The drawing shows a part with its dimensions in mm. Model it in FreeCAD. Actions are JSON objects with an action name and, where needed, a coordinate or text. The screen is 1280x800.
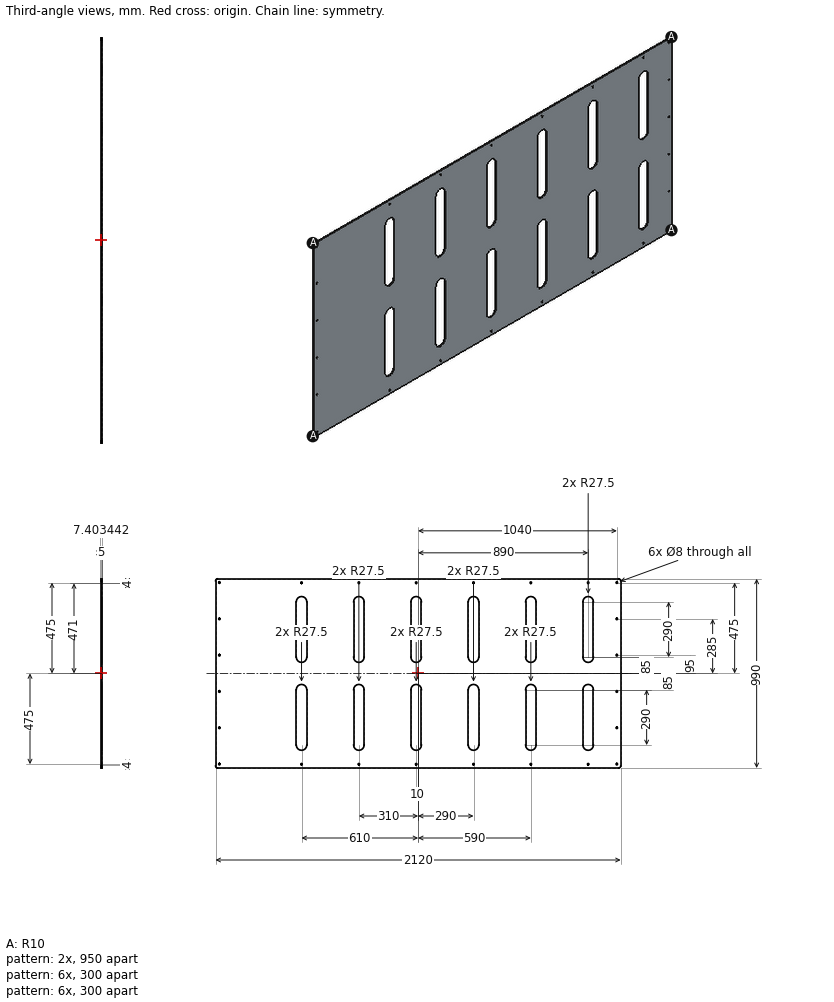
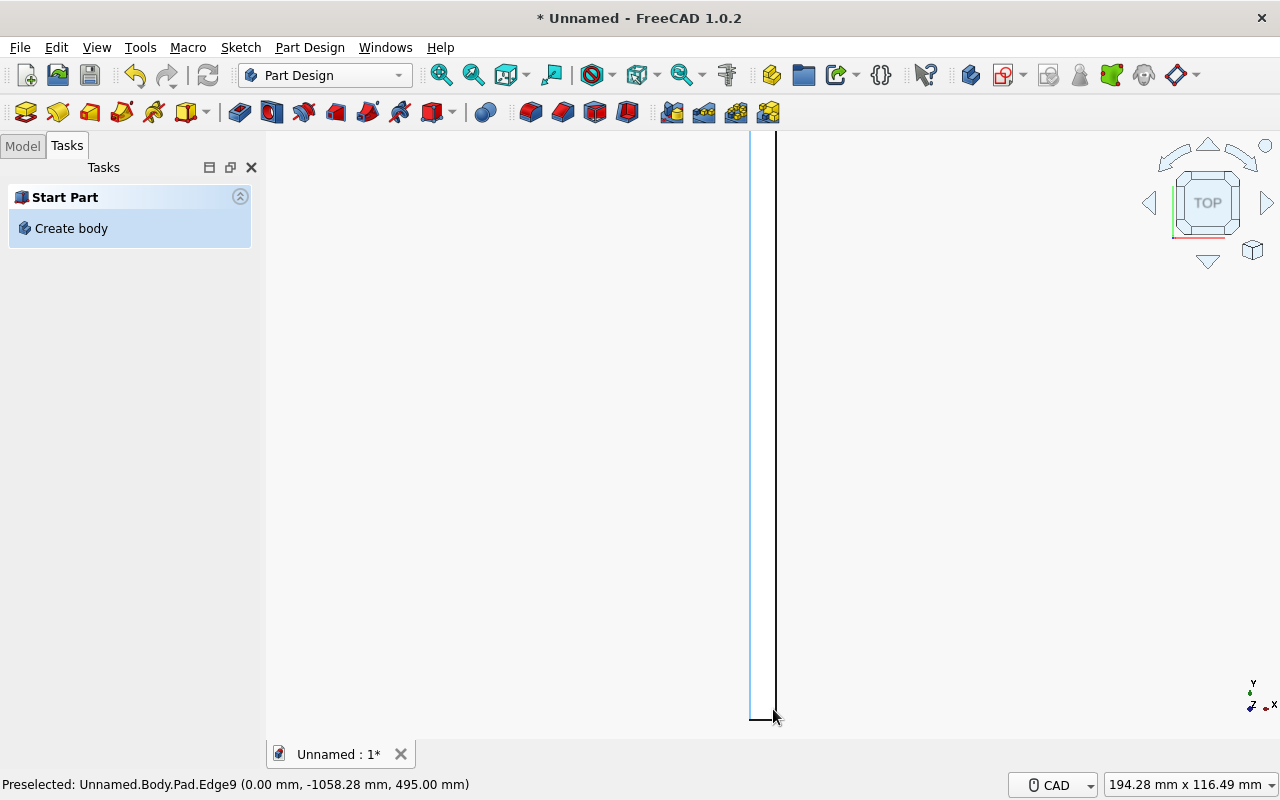
{"action": "left_click", "coordinate": [442, 76]}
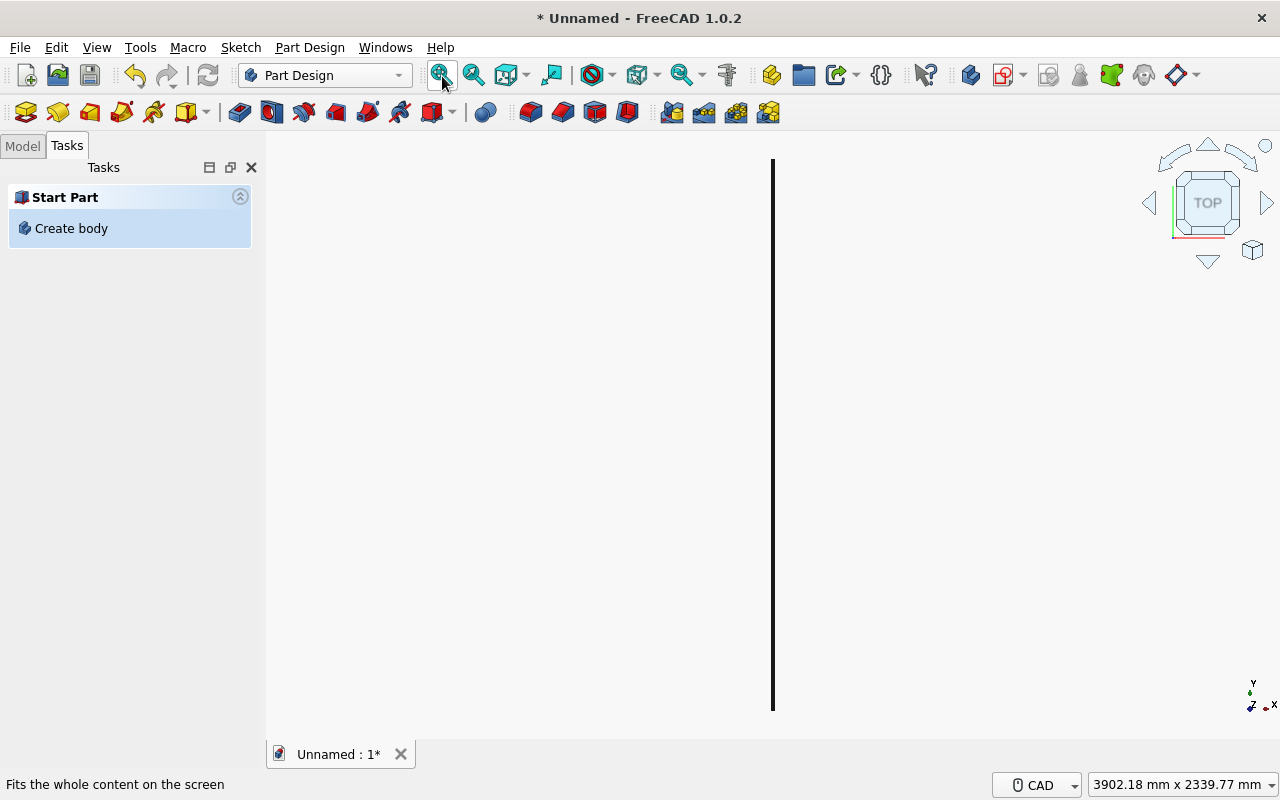
{"action": "key", "text": "1"}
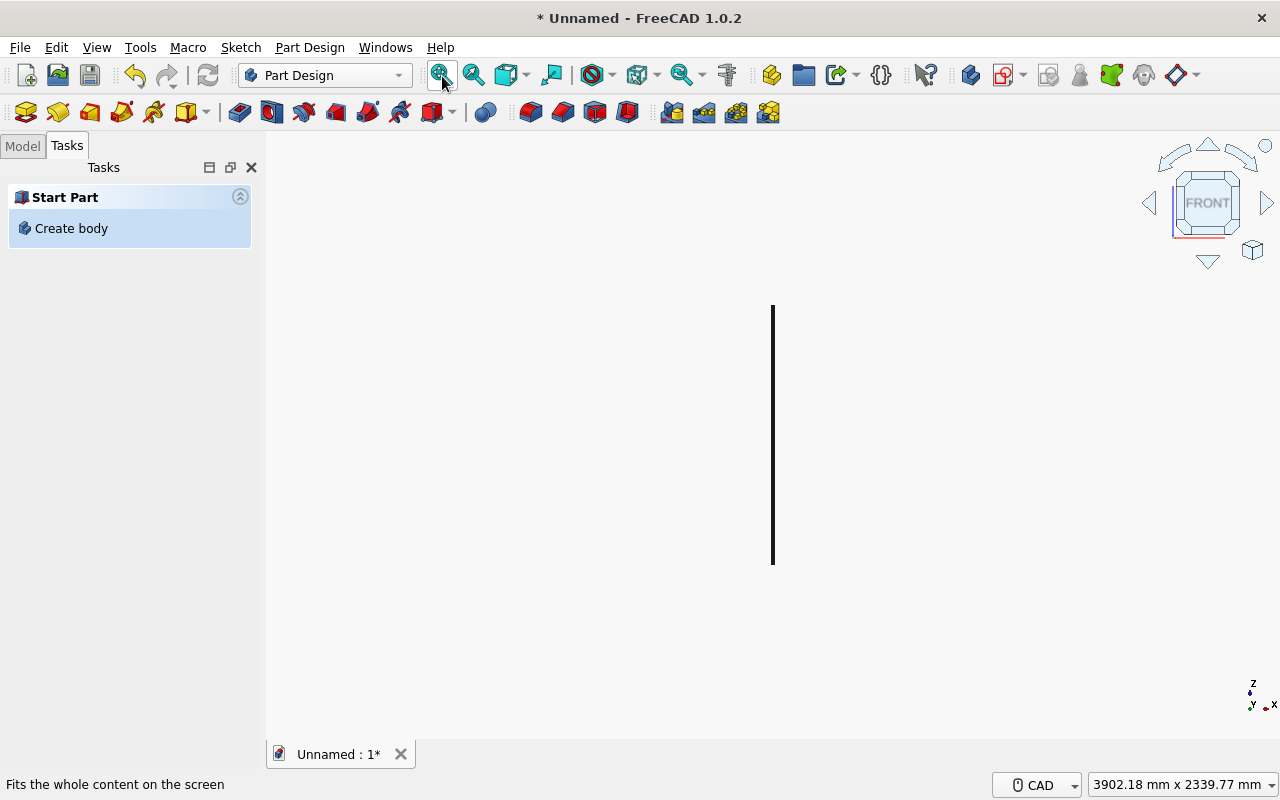
{"action": "key", "text": "v f"}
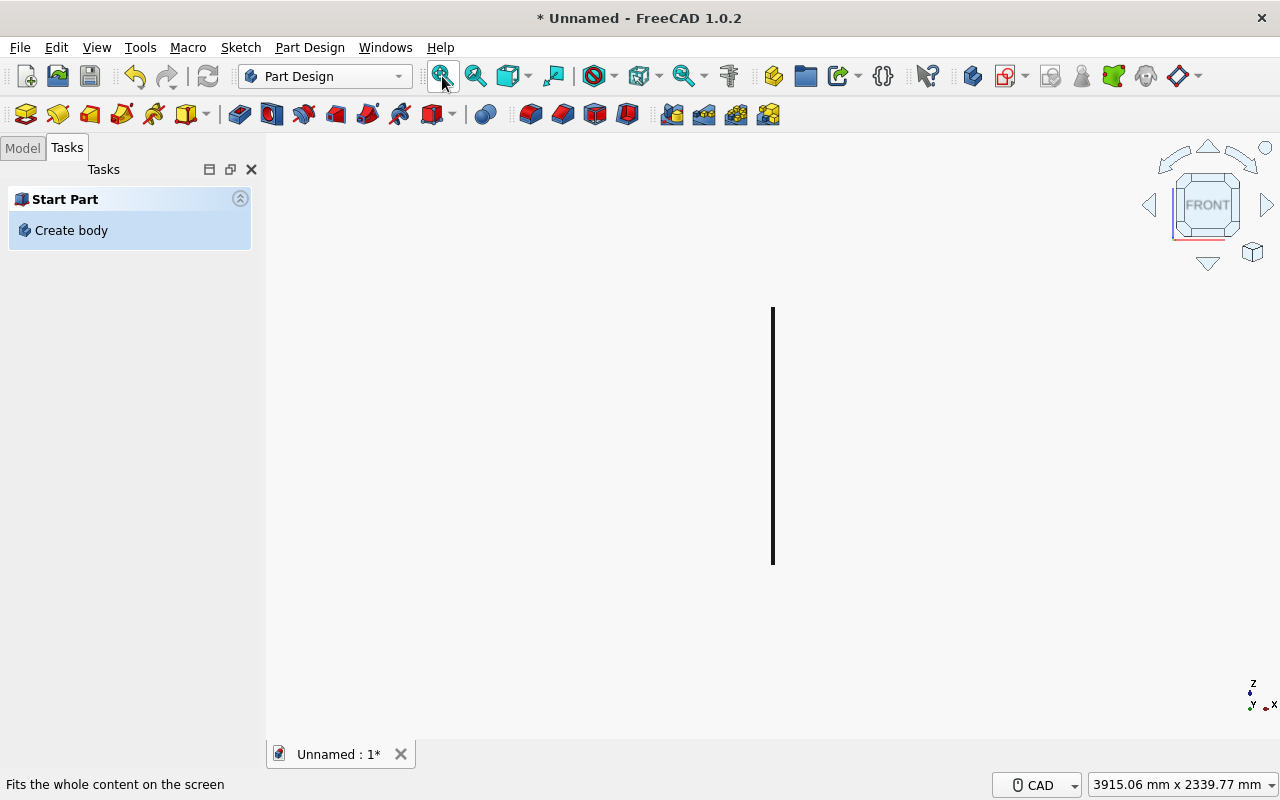
{"action": "scroll", "coordinate": [773, 563], "scroll_direction": "up", "scroll_amount": 15}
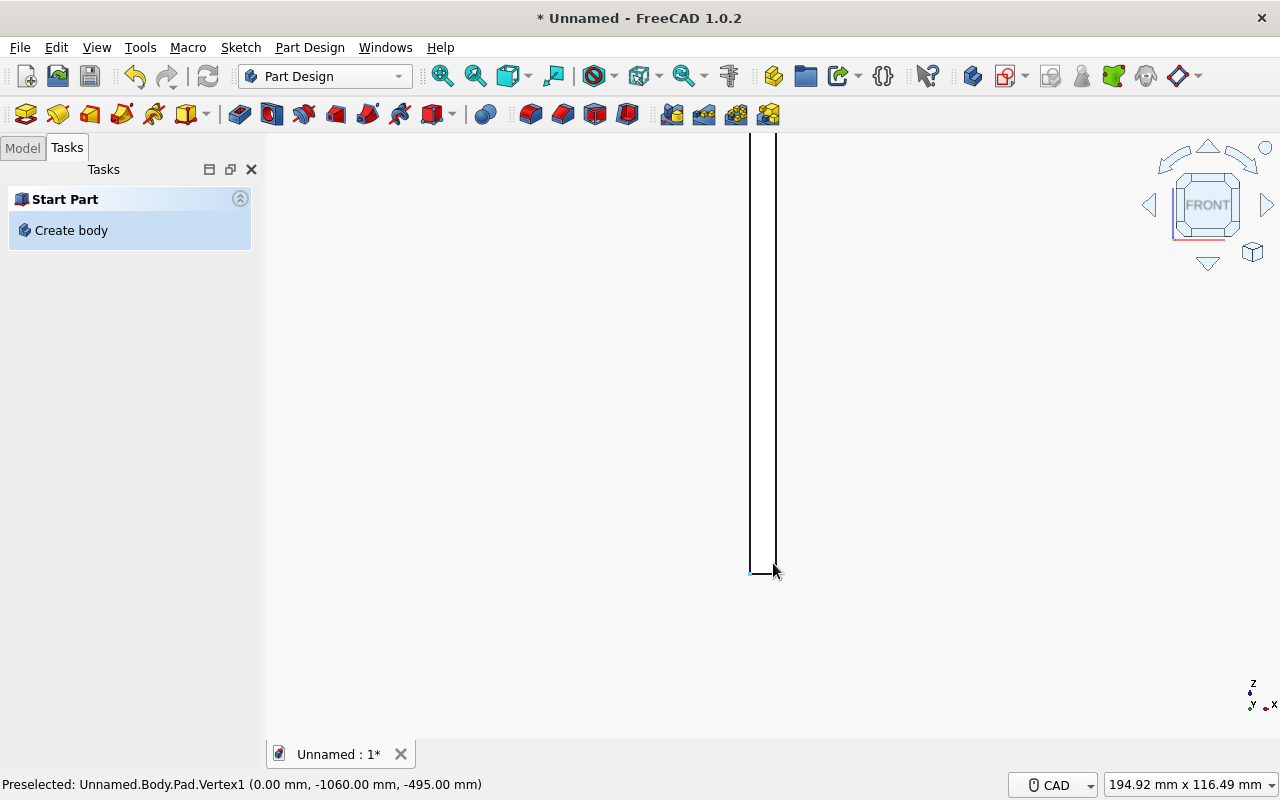
{"action": "left_click", "coordinate": [763, 573]}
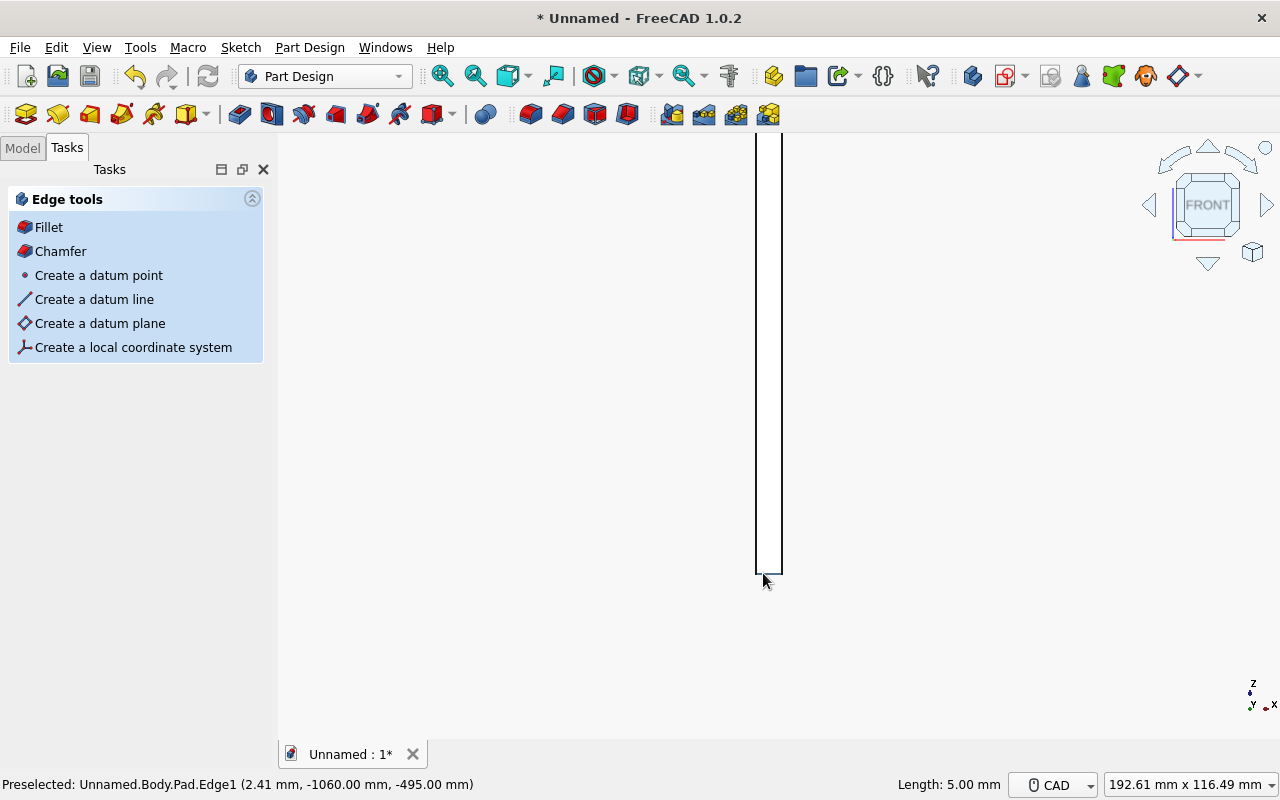
{"action": "left_click", "coordinate": [444, 76]}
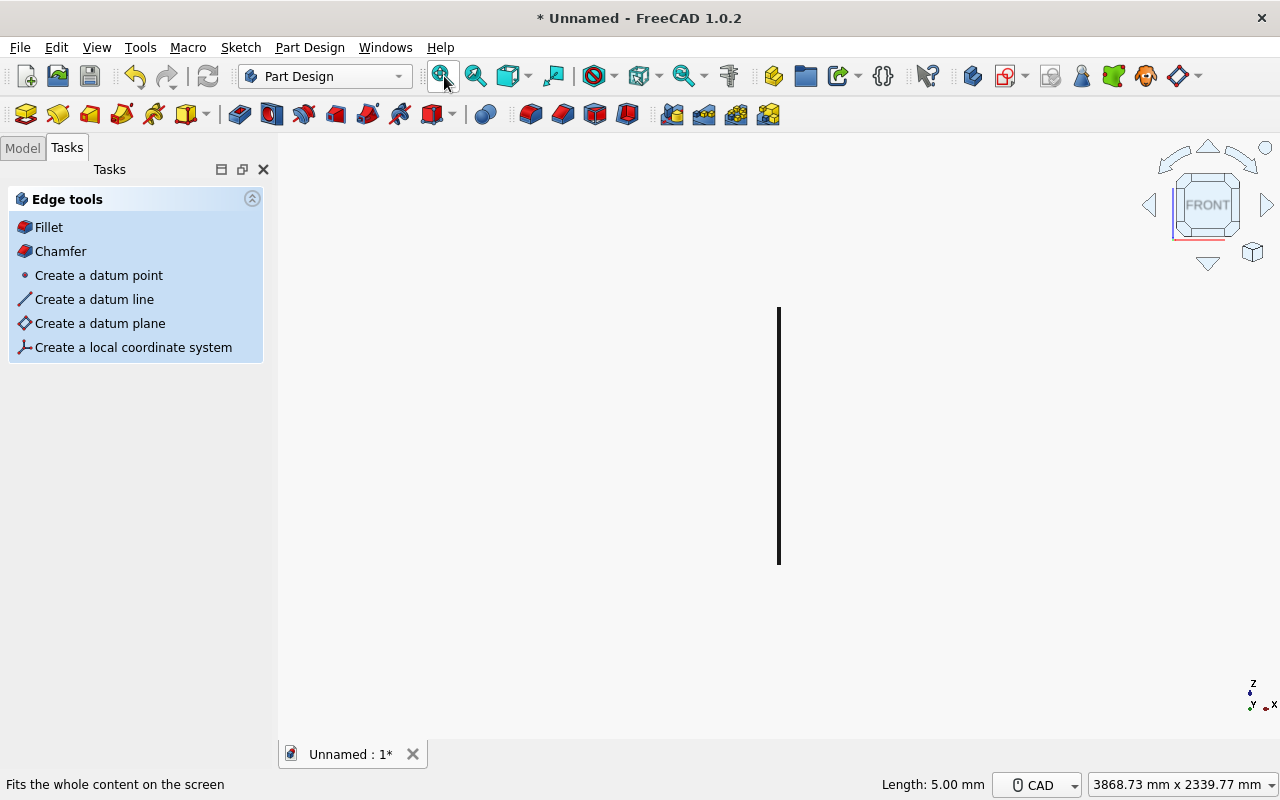
{"action": "key", "text": "3"}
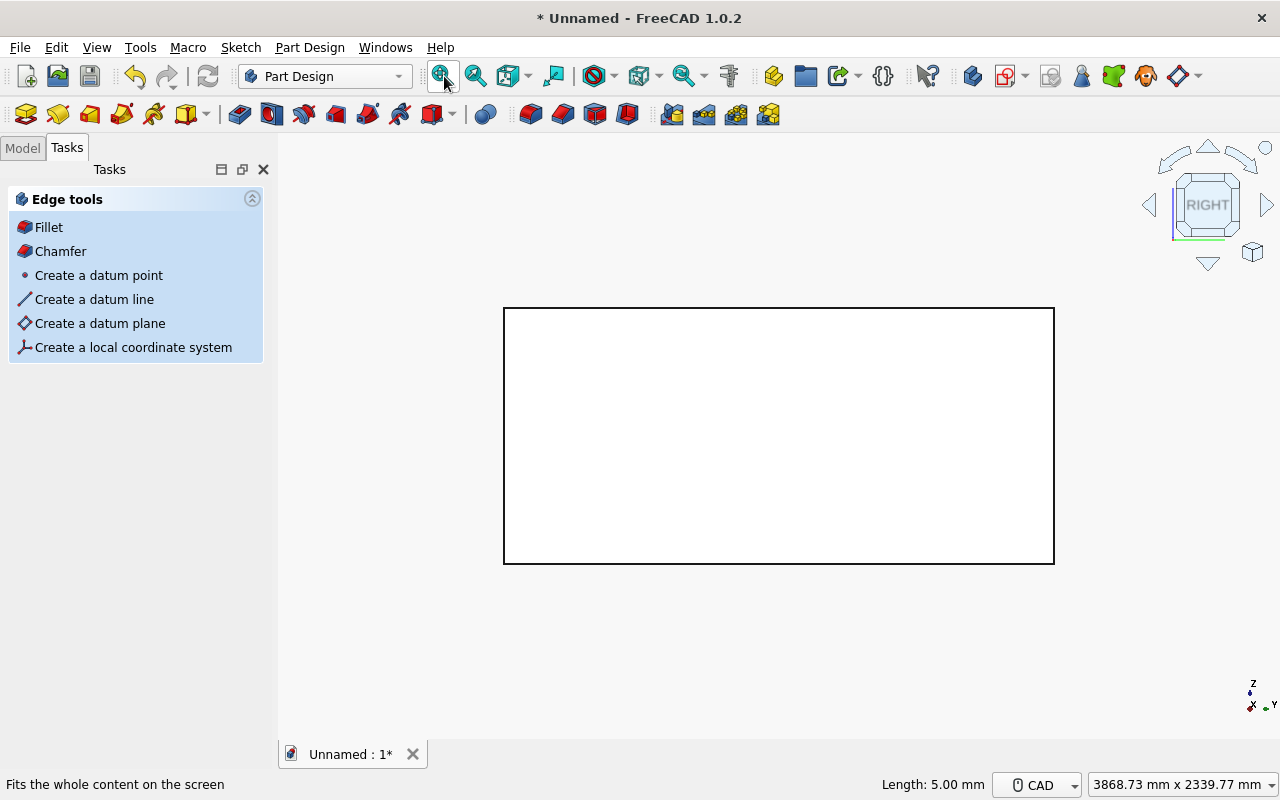
{"action": "scroll", "coordinate": [504, 307], "scroll_direction": "up", "scroll_amount": 15}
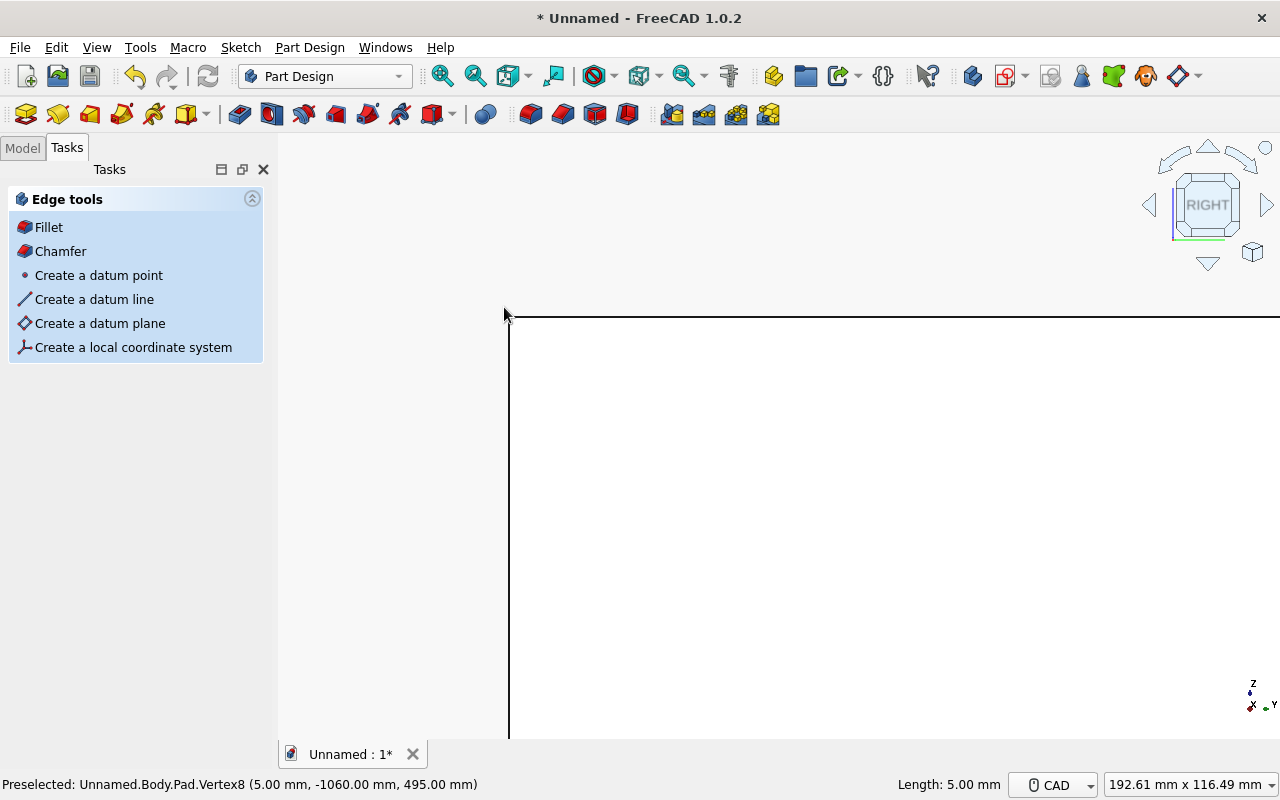
{"action": "left_click", "coordinate": [444, 76]}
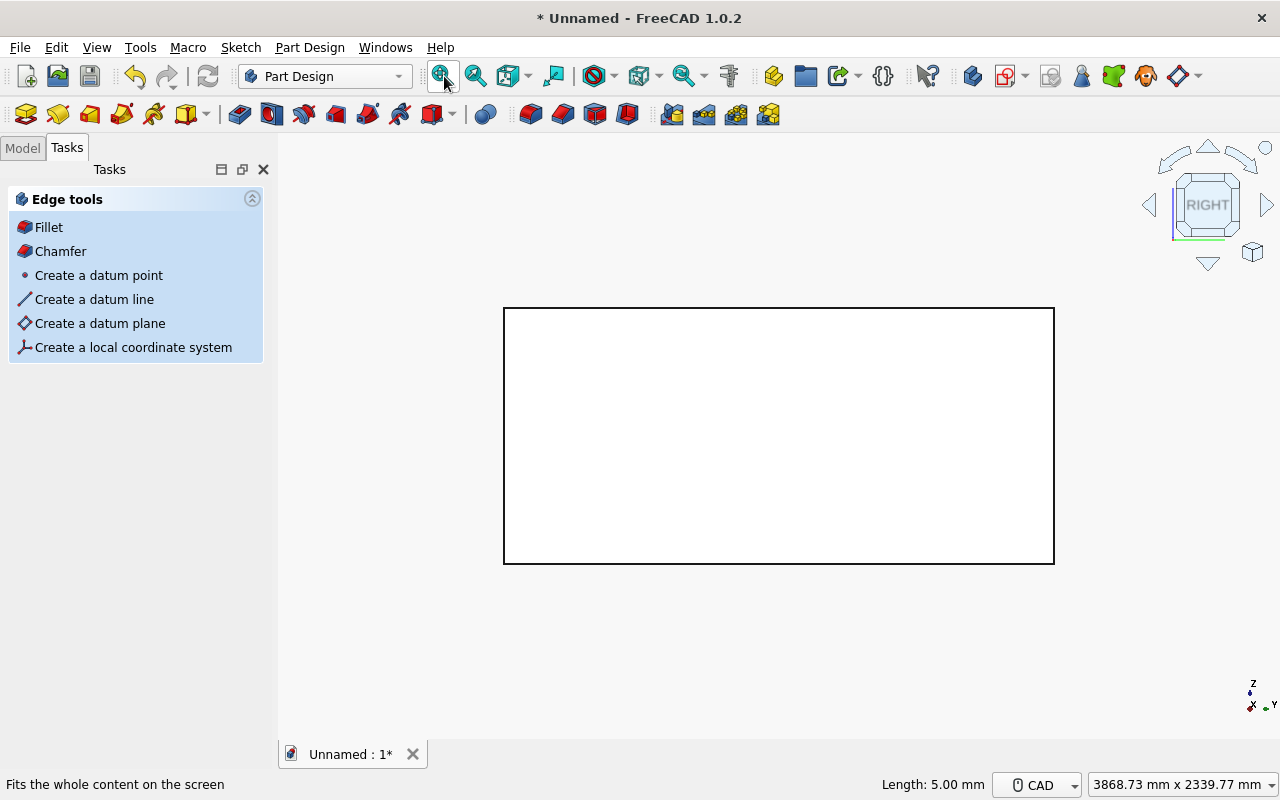
{"action": "key", "text": "5"}